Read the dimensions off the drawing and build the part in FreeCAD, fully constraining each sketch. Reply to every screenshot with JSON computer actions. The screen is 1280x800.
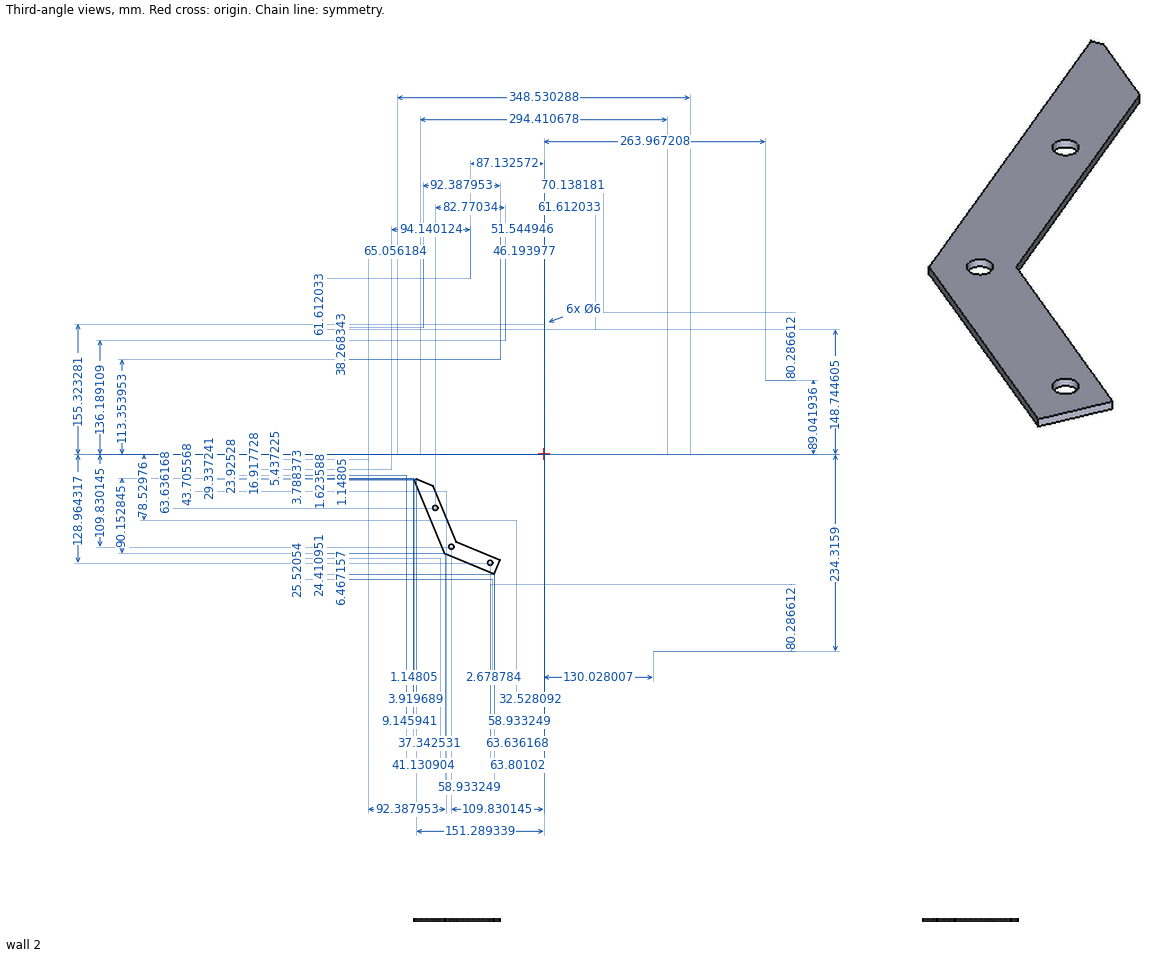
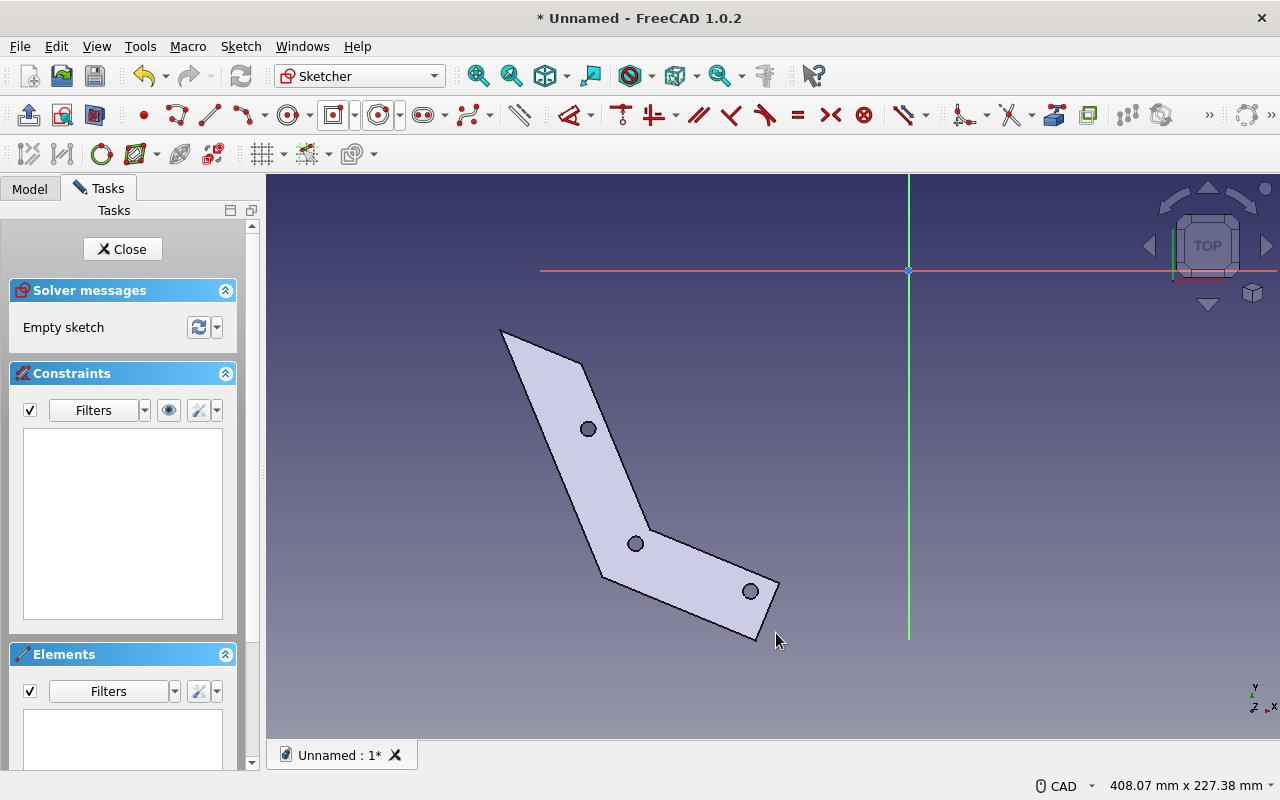
{"action": "left_click", "coordinate": [177, 116]}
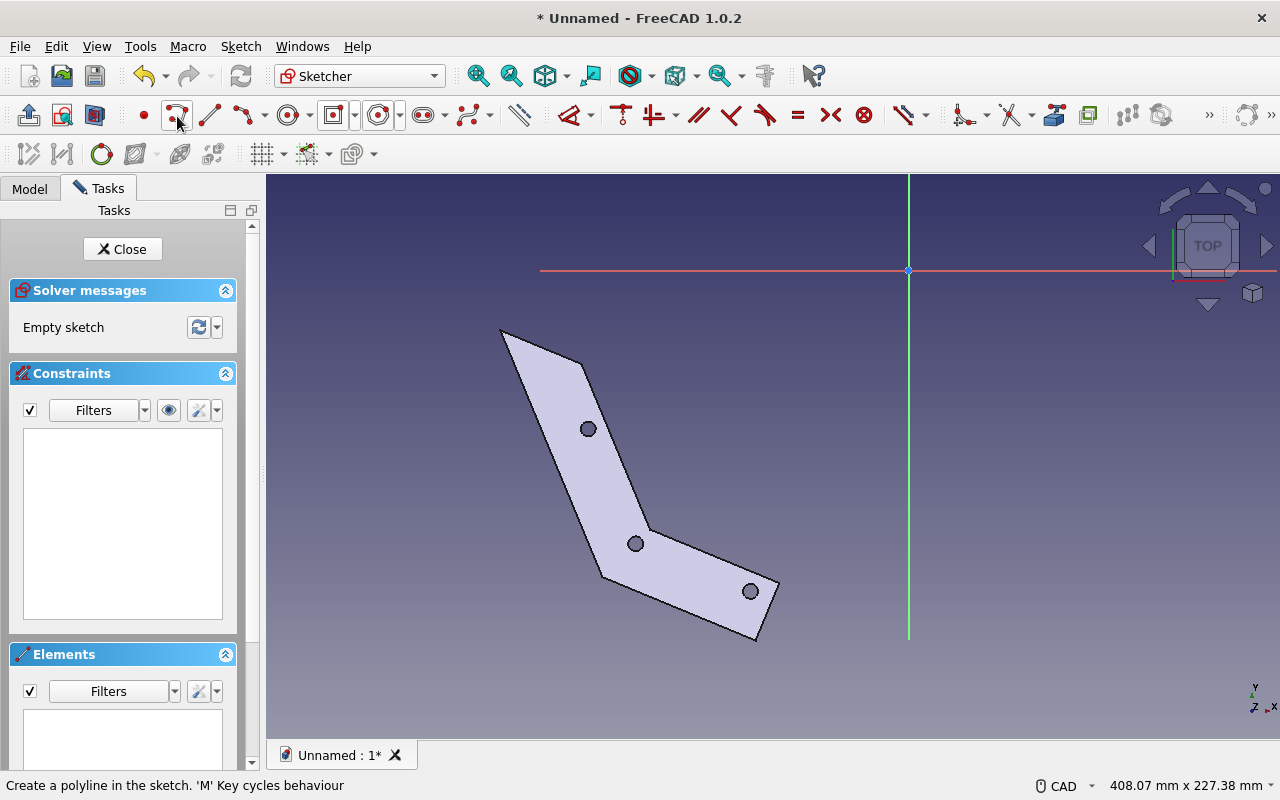
{"action": "left_click", "coordinate": [762, 624]}
{"action": "left_click", "coordinate": [616, 564]}
{"action": "left_click", "coordinate": [523, 340]}
{"action": "left_click", "coordinate": [500, 330]}
{"action": "left_click", "coordinate": [602, 577]}
{"action": "left_click", "coordinate": [756, 641]}
{"action": "left_click", "coordinate": [762, 625]}
{"action": "key", "text": "Escape"}
{"action": "key", "text": "Escape"}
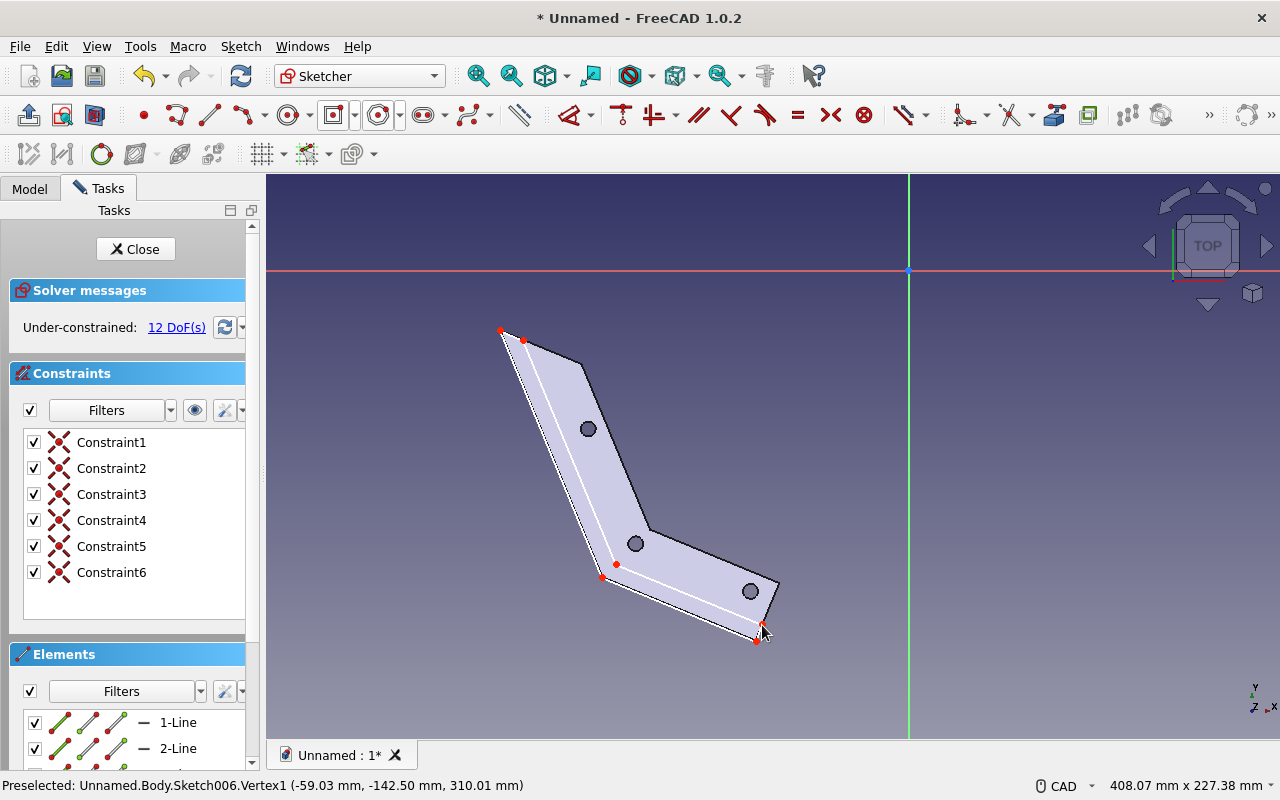
{"action": "left_click", "coordinate": [568, 116]}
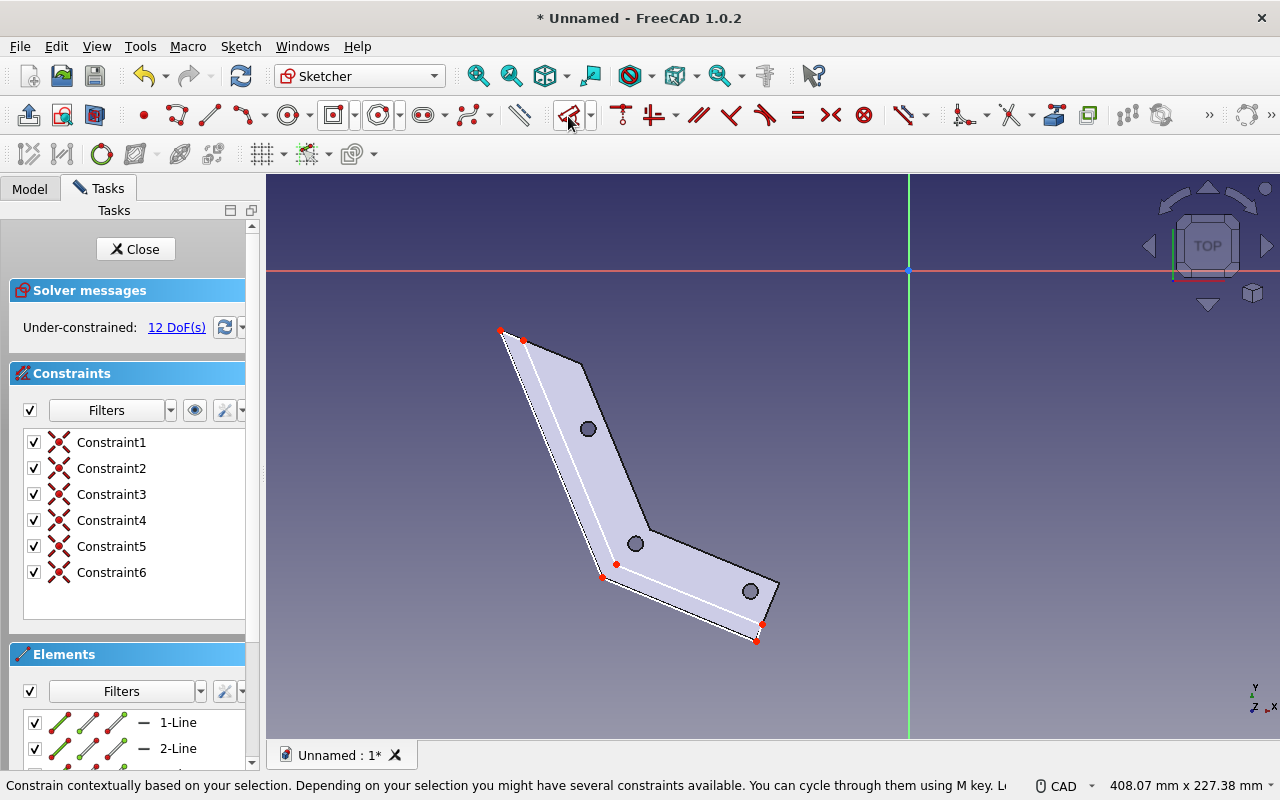
{"action": "left_click", "coordinate": [500, 331]}
{"action": "left_click", "coordinate": [466, 301]}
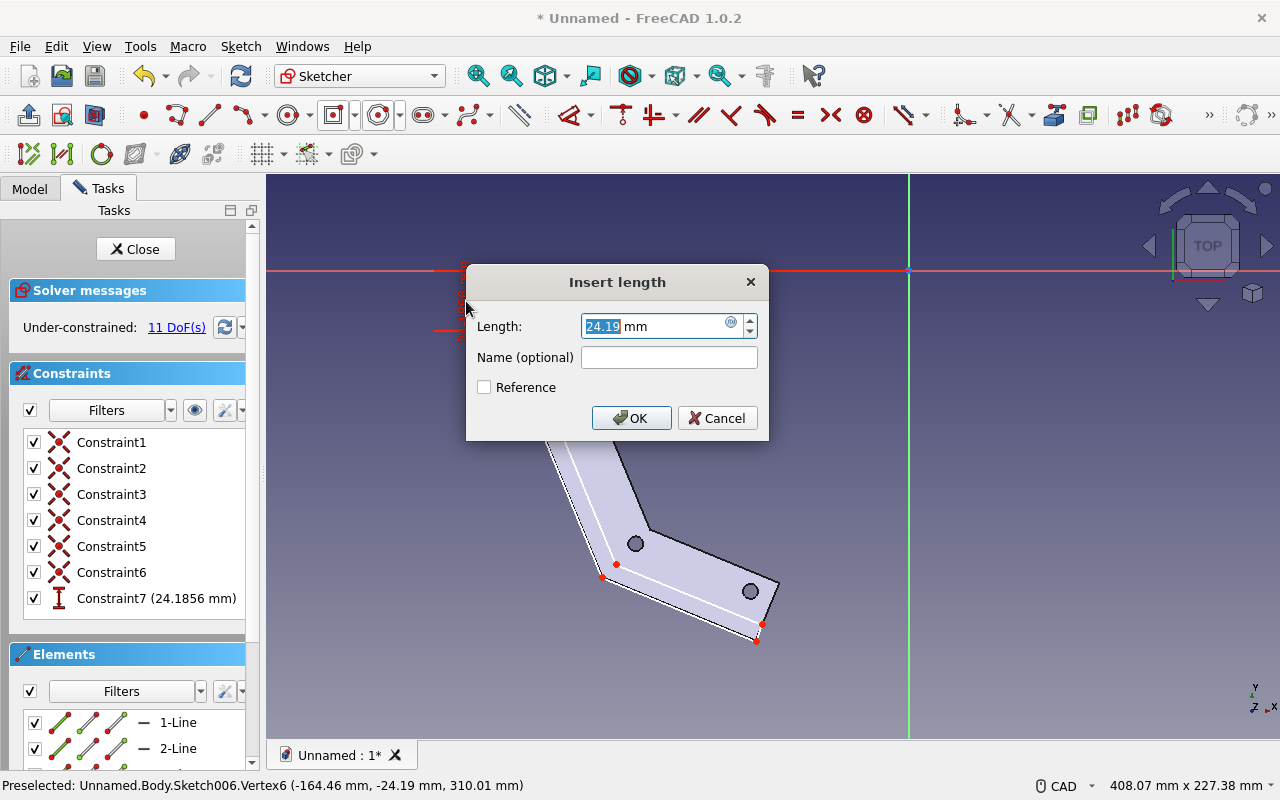
{"action": "type", "text": "23.92528"}
{"action": "key", "text": "Return"}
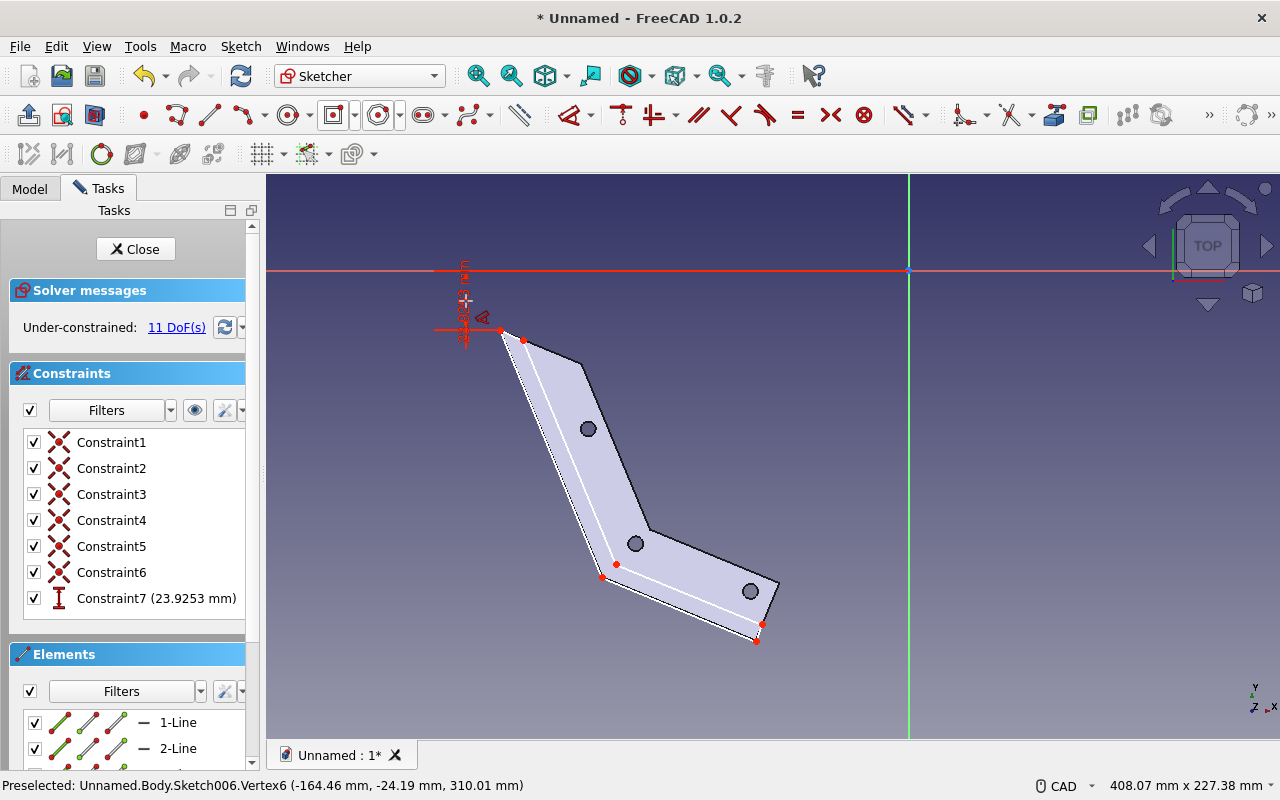
{"action": "scroll", "coordinate": [514, 337], "scroll_direction": "up", "scroll_amount": 3}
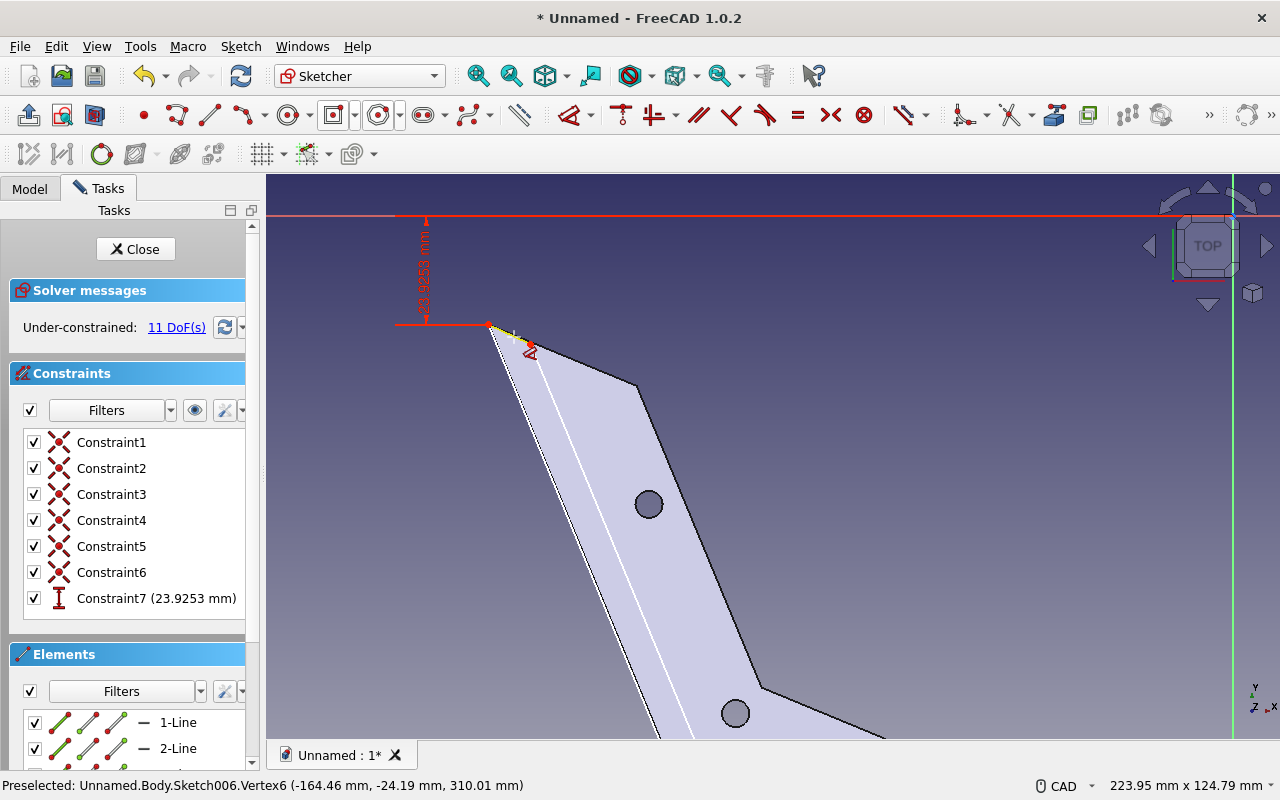
{"action": "left_click", "coordinate": [513, 336]}
{"action": "left_click", "coordinate": [509, 291]}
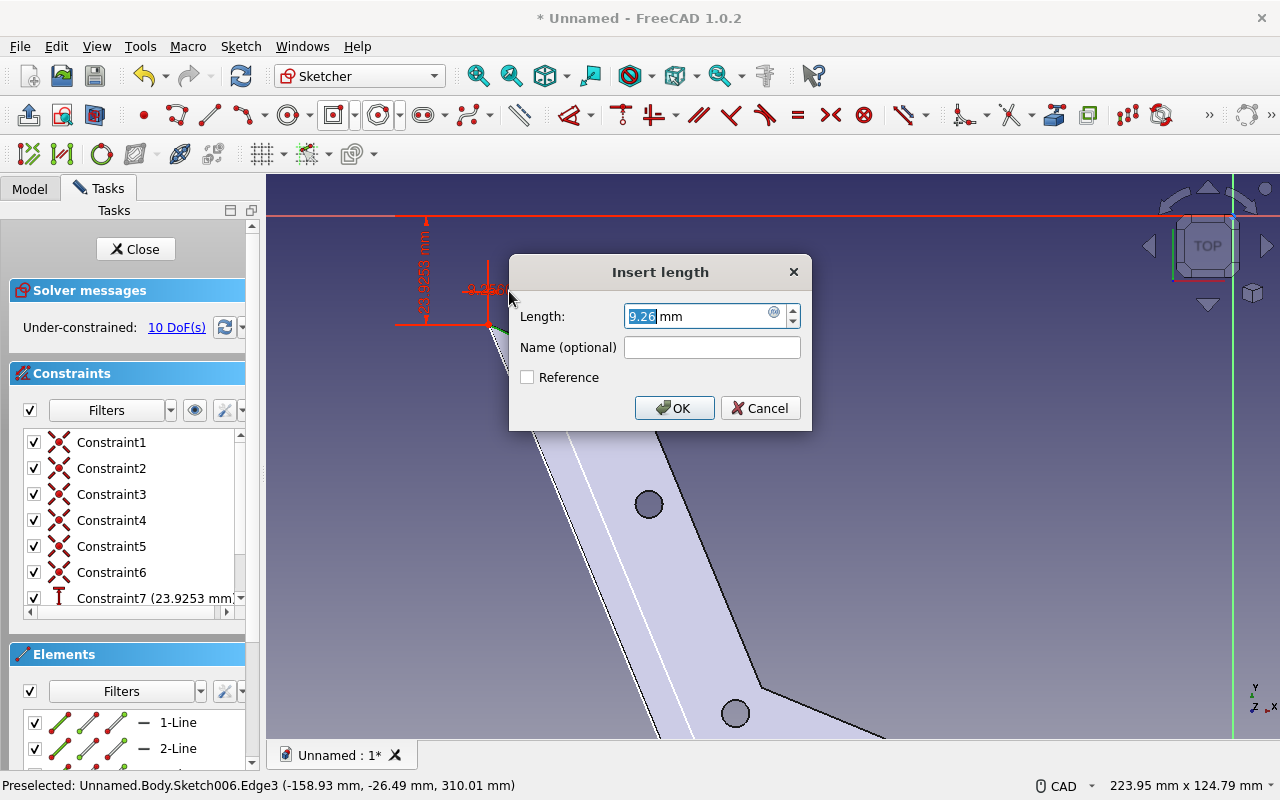
{"action": "type", "text": "9.145941"}
{"action": "key", "text": "Return"}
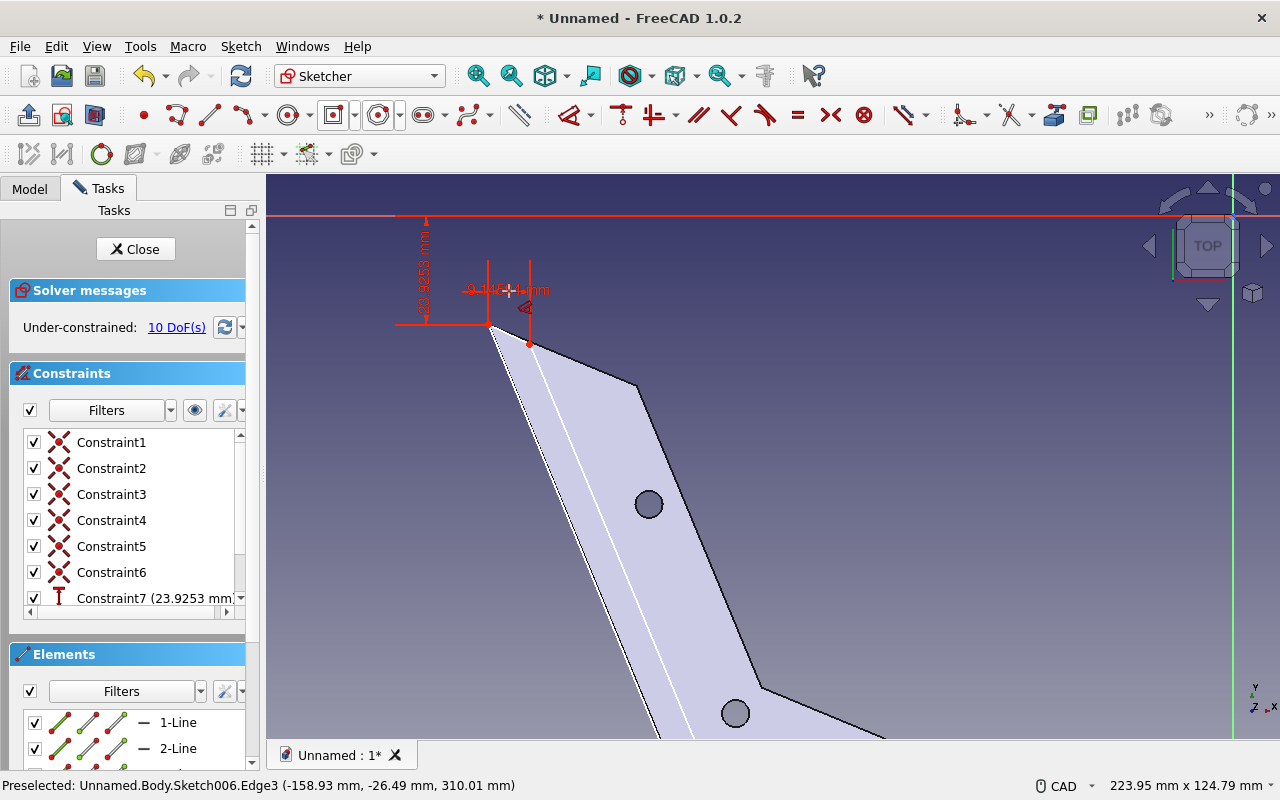
{"action": "scroll", "coordinate": [517, 338], "scroll_direction": "up", "scroll_amount": 5}